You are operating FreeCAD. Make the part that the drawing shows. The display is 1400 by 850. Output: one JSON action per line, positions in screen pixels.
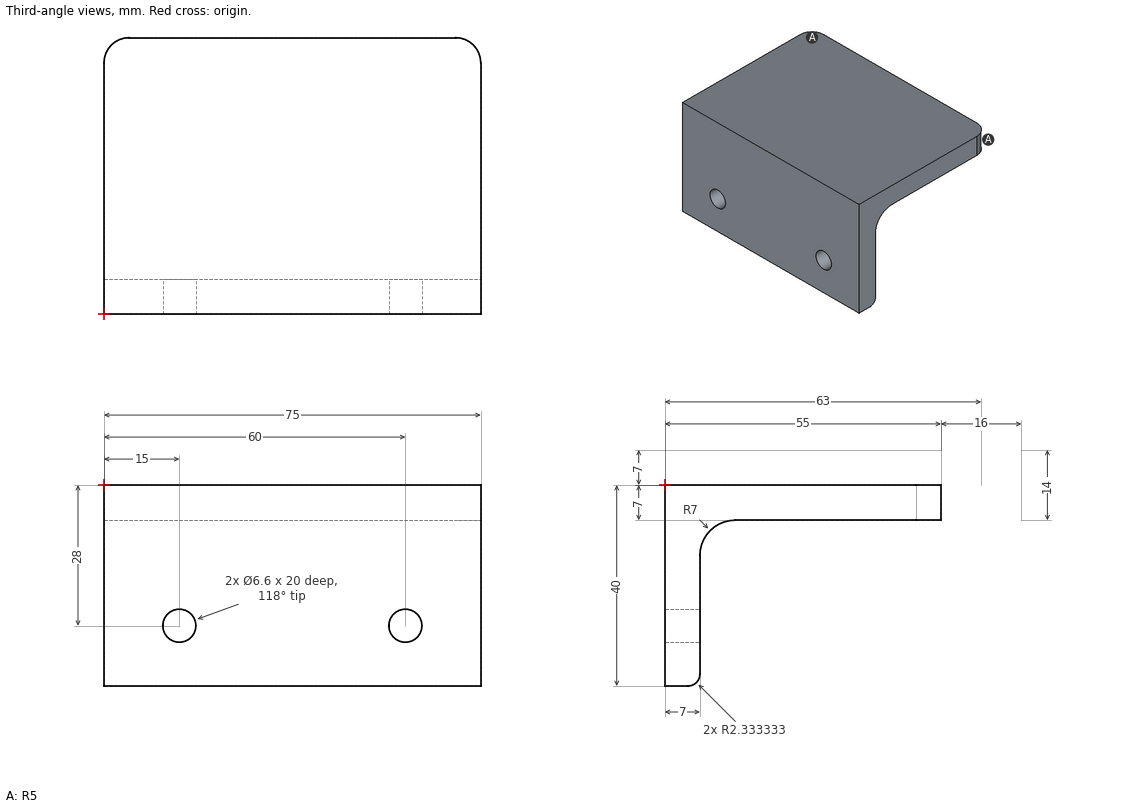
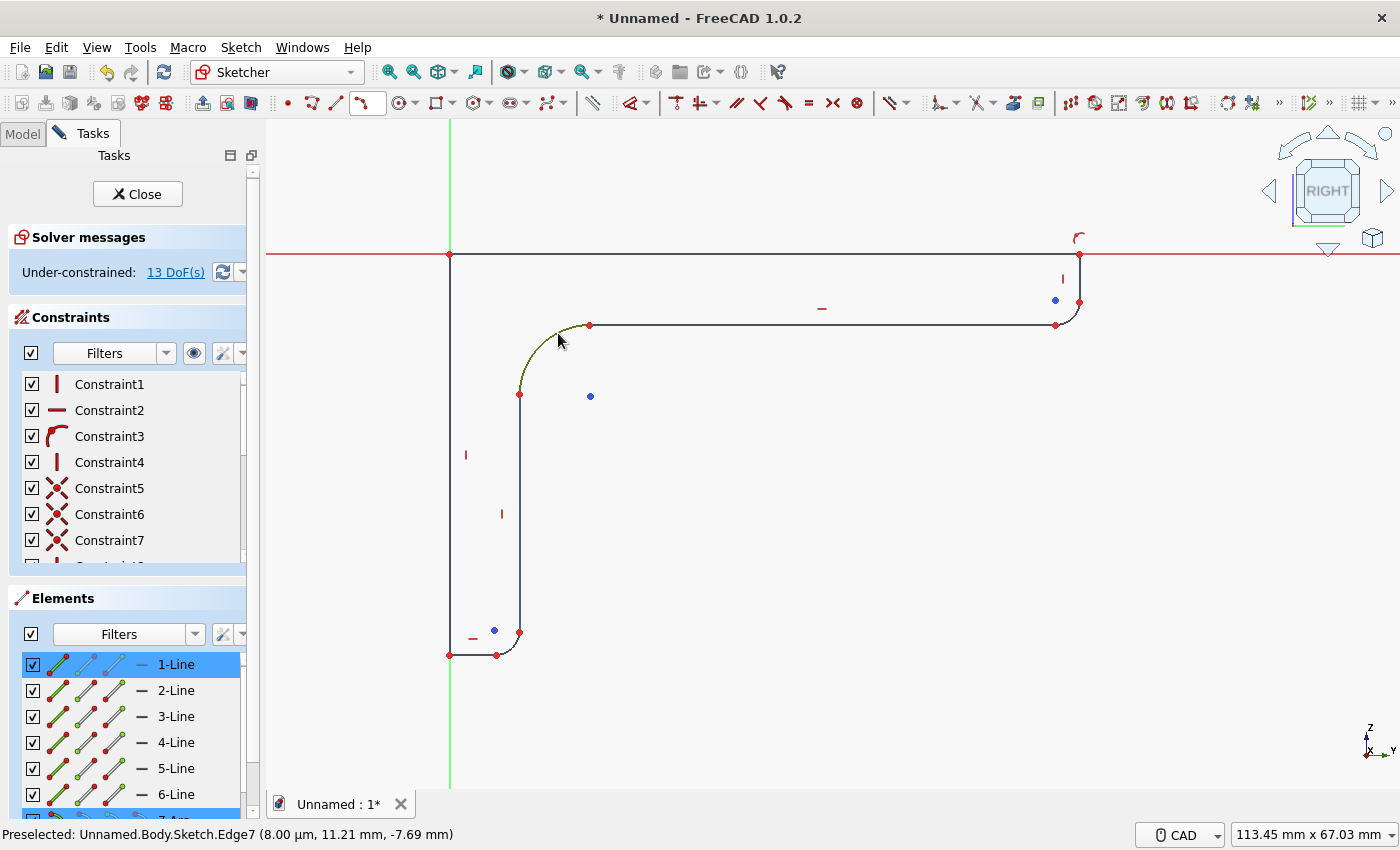
{"action": "left_click", "coordinate": [786, 104]}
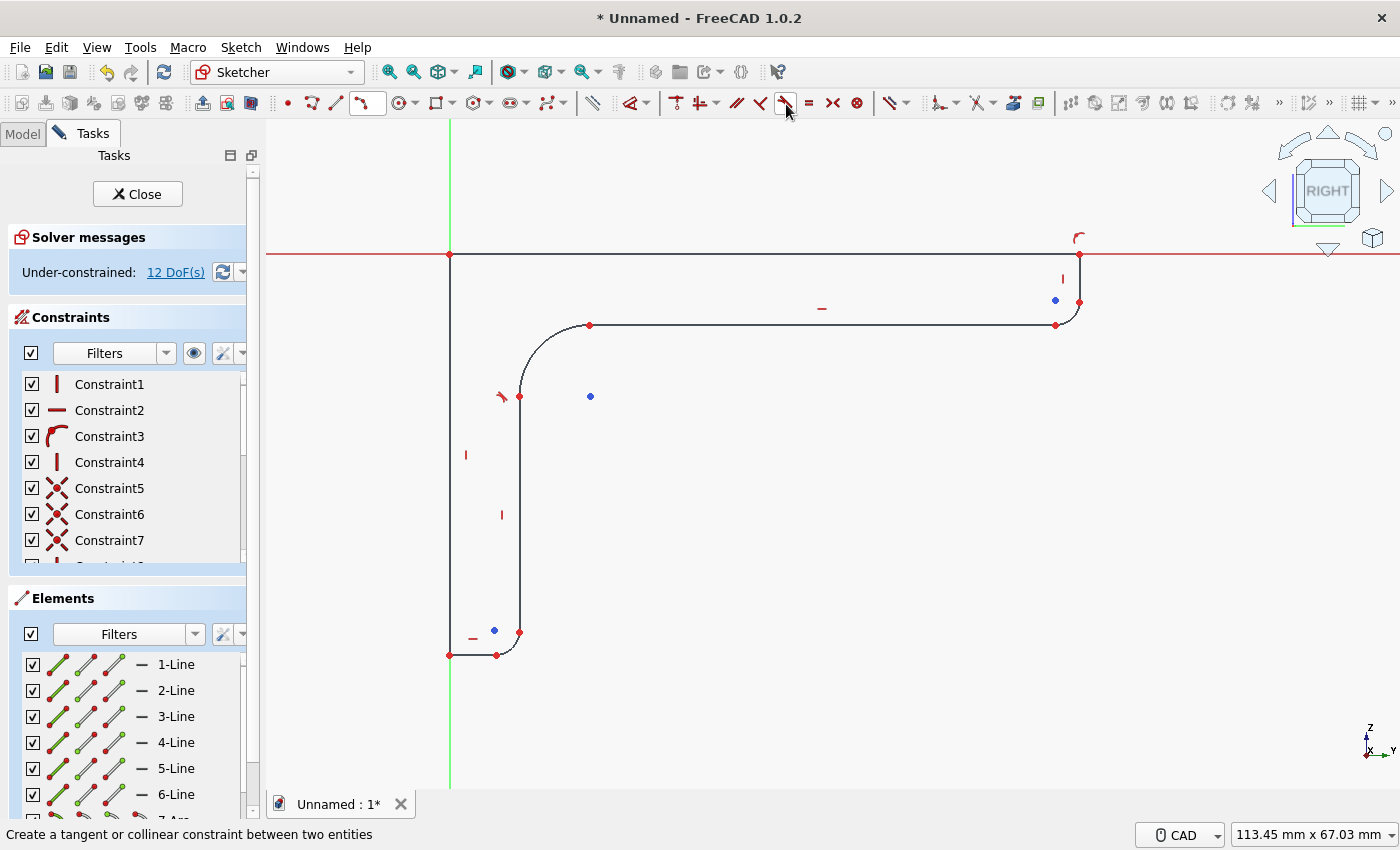
{"action": "left_click", "coordinate": [520, 561]}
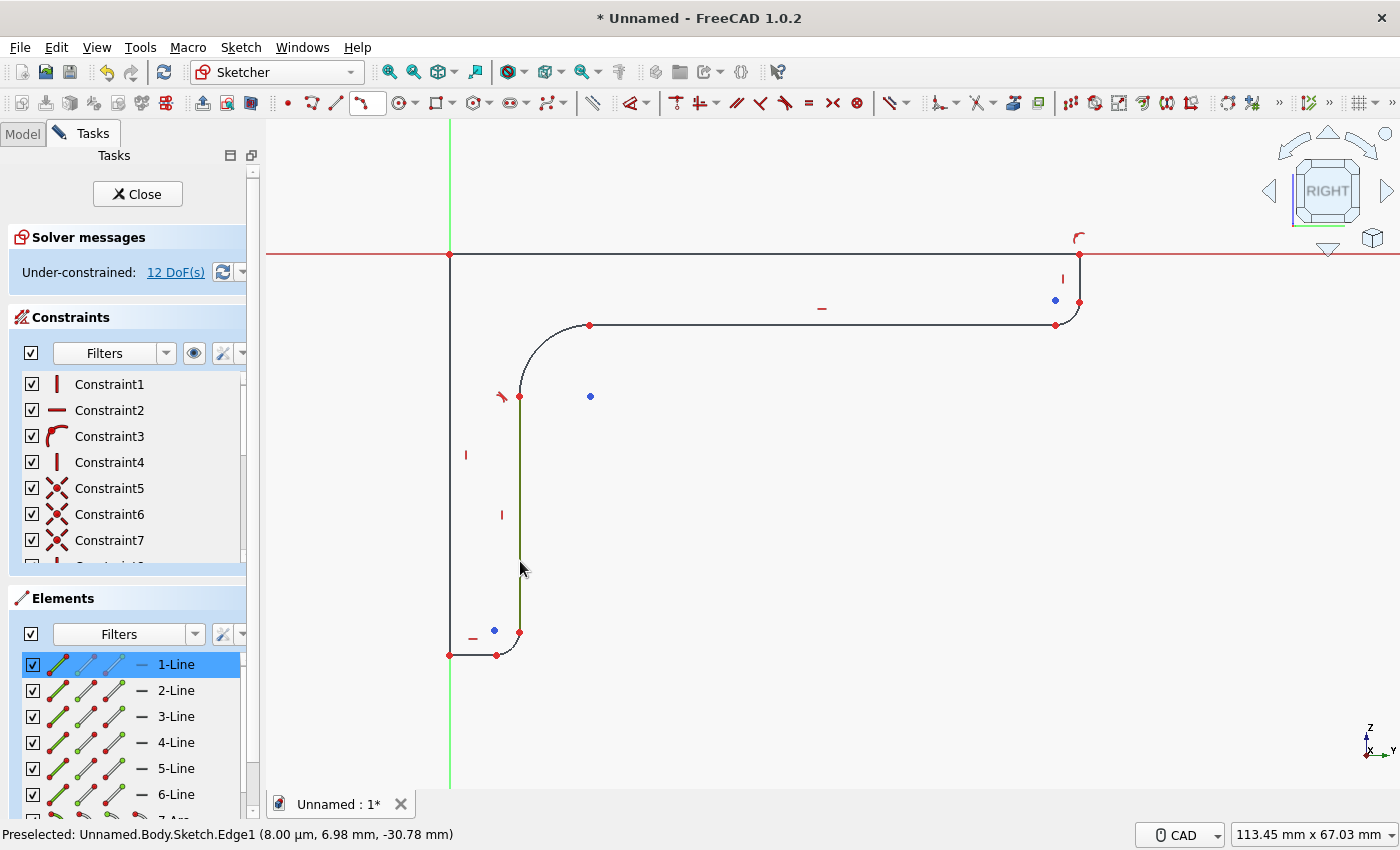
{"action": "scroll", "coordinate": [507, 652], "scroll_direction": "up", "scroll_amount": 2}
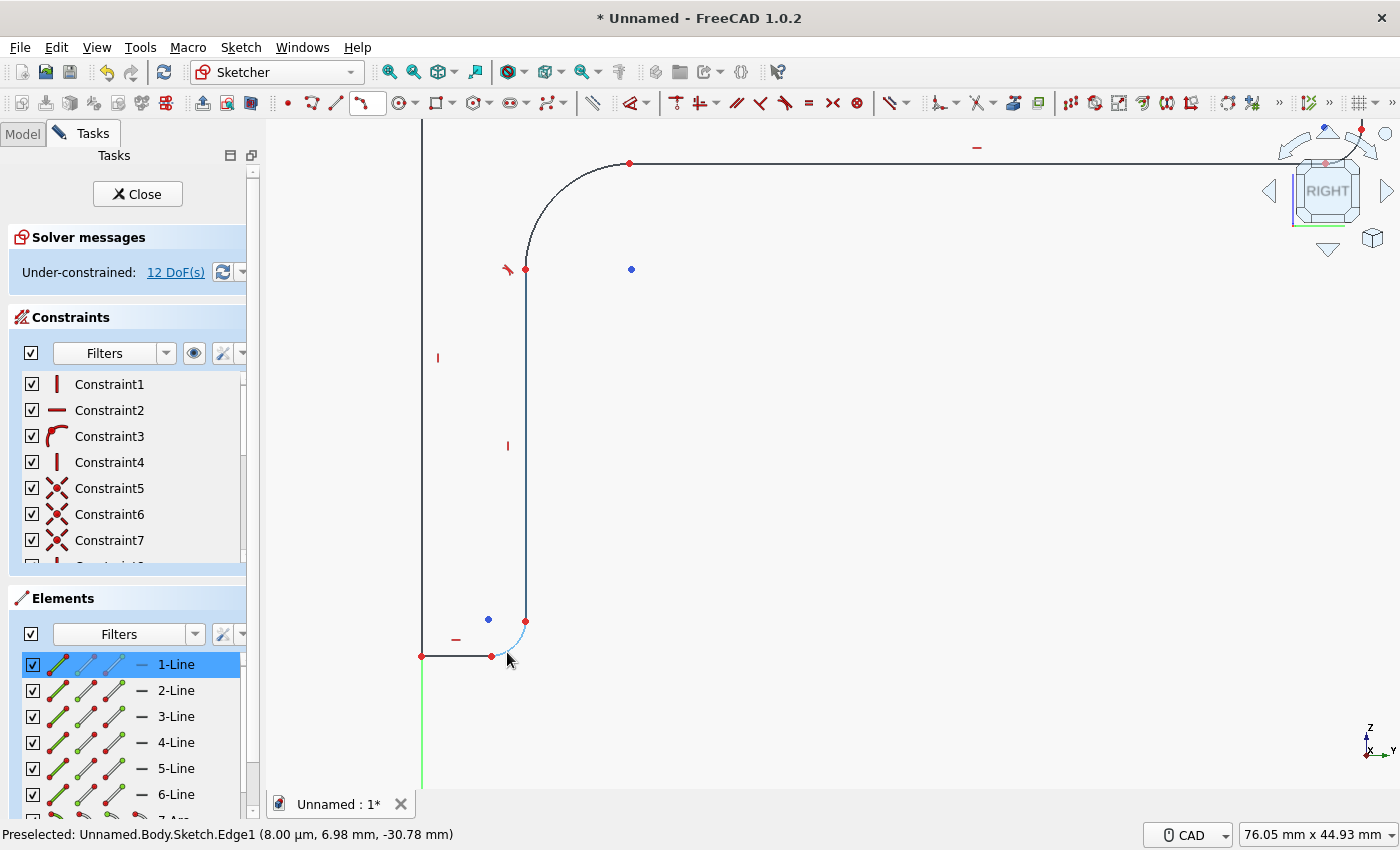
{"action": "left_click", "coordinate": [507, 652]}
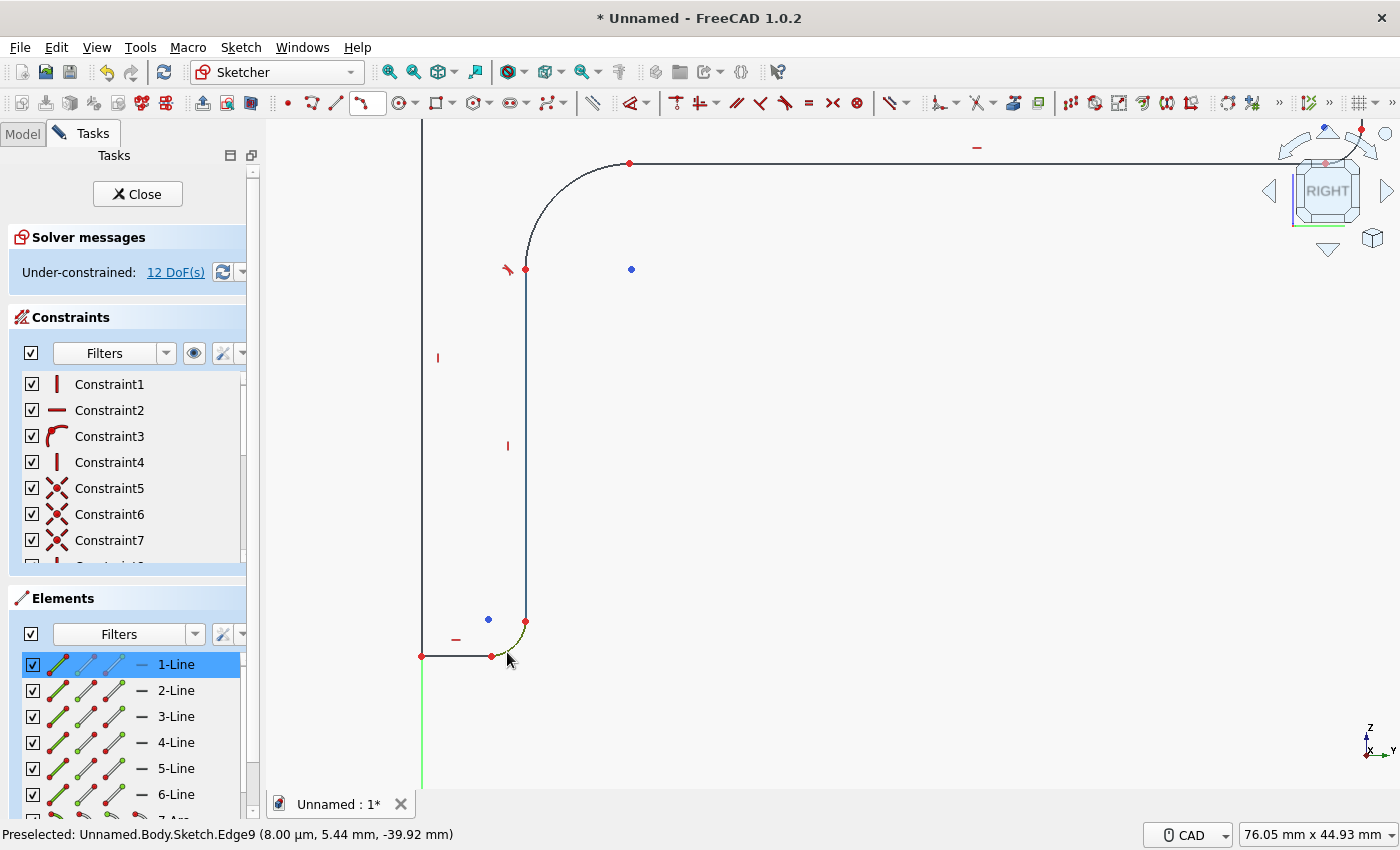
{"action": "key", "text": "t"}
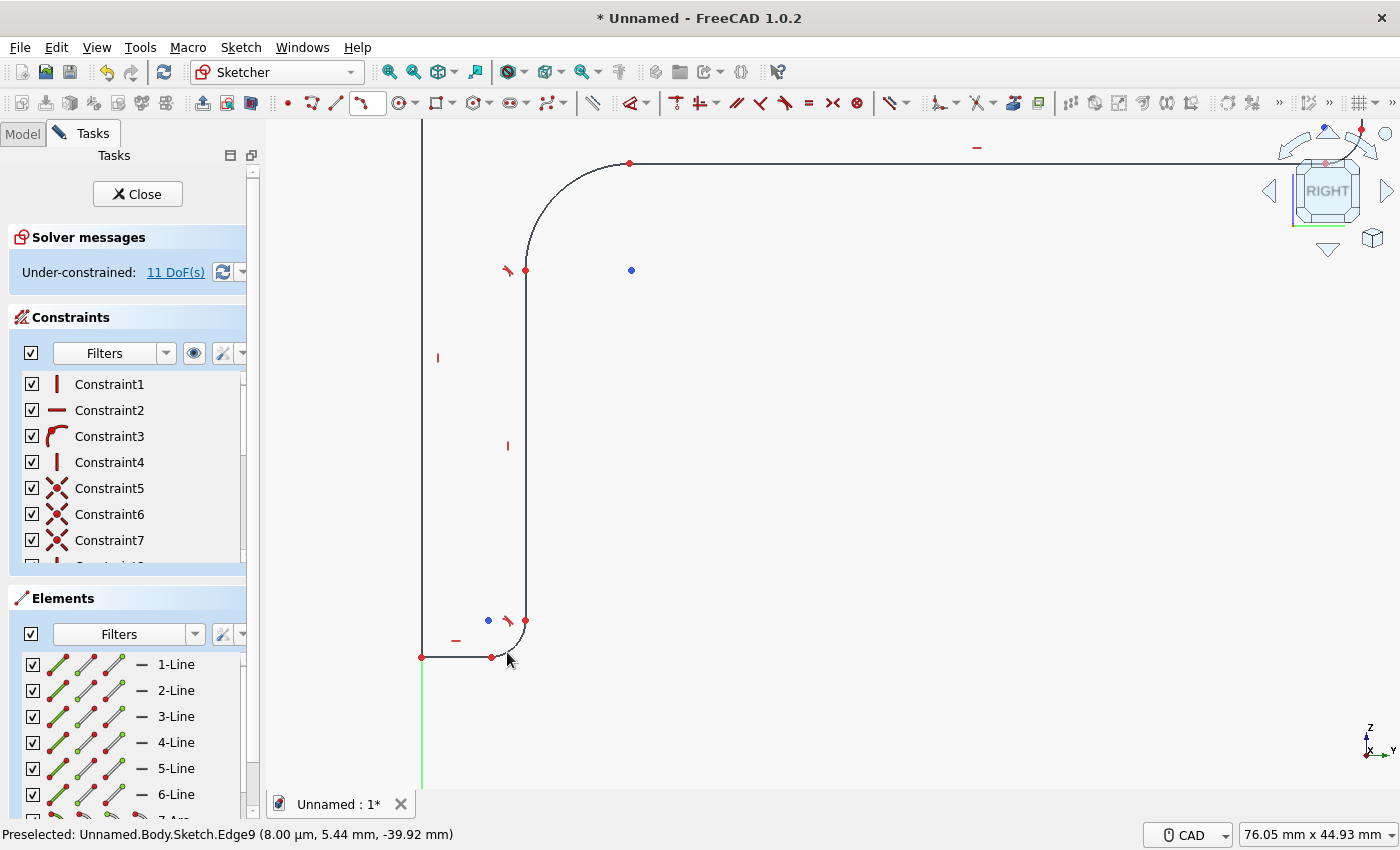
{"action": "left_click", "coordinate": [839, 164]}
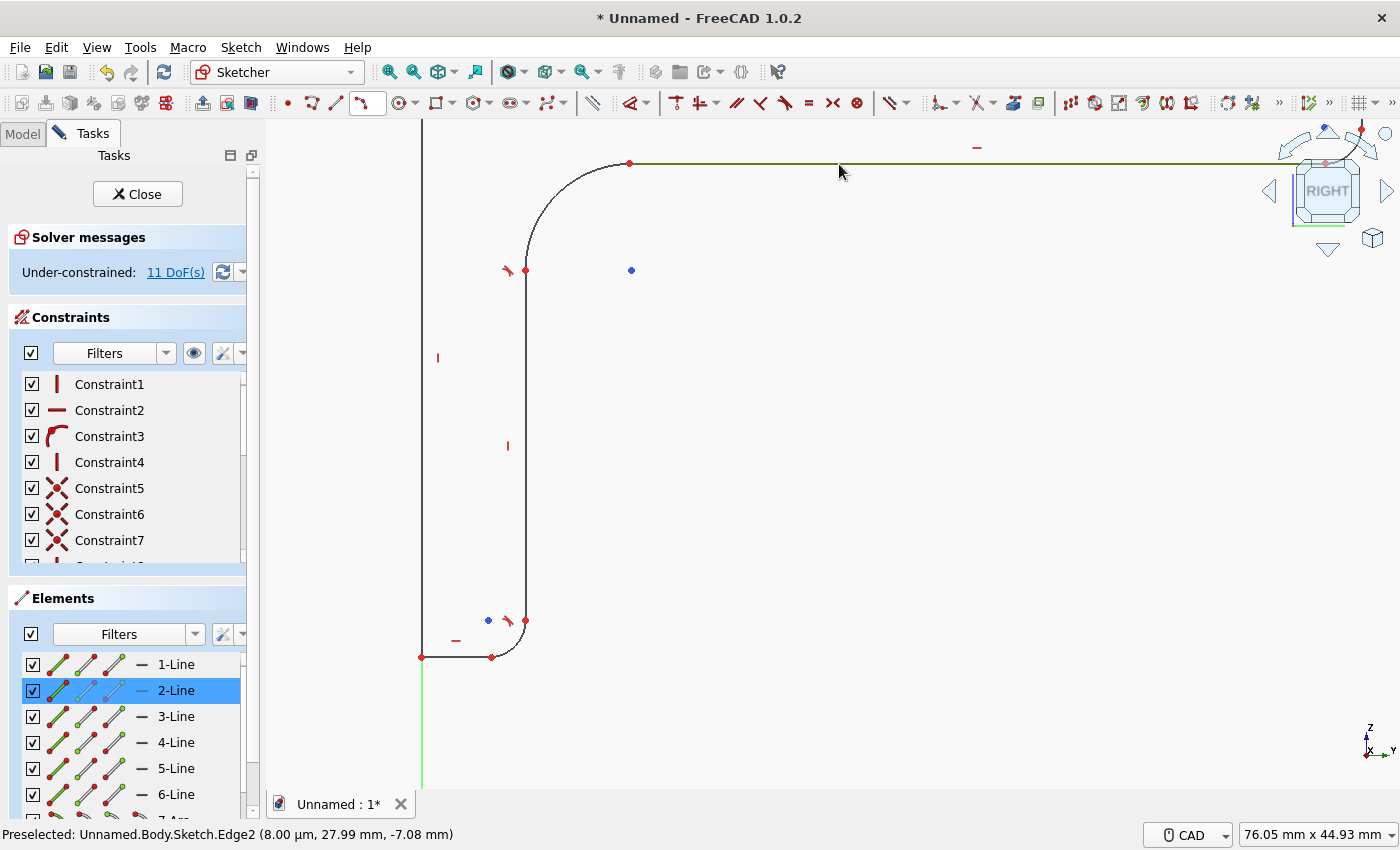
{"action": "left_click", "coordinate": [582, 176]}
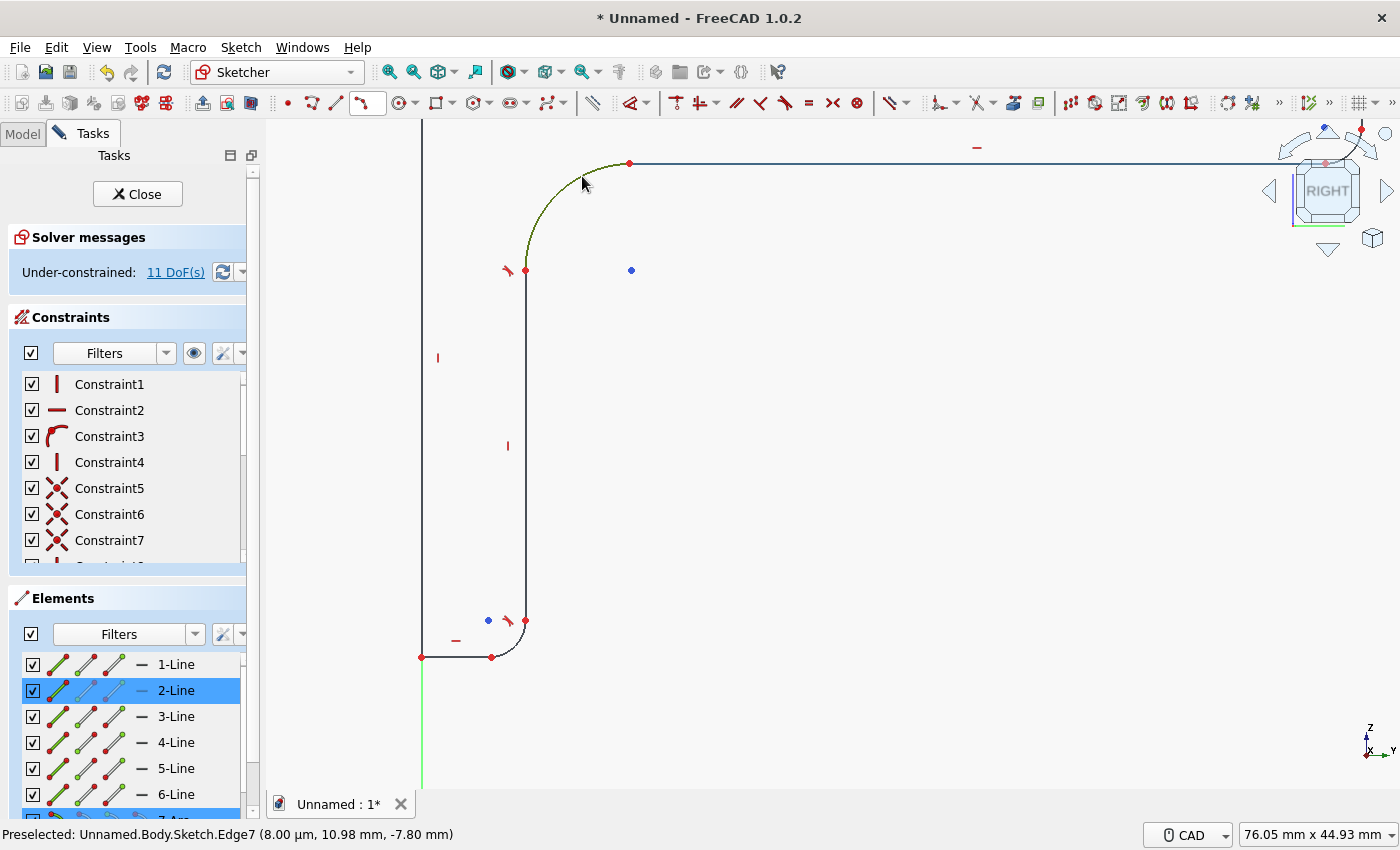
{"action": "left_click", "coordinate": [786, 104]}